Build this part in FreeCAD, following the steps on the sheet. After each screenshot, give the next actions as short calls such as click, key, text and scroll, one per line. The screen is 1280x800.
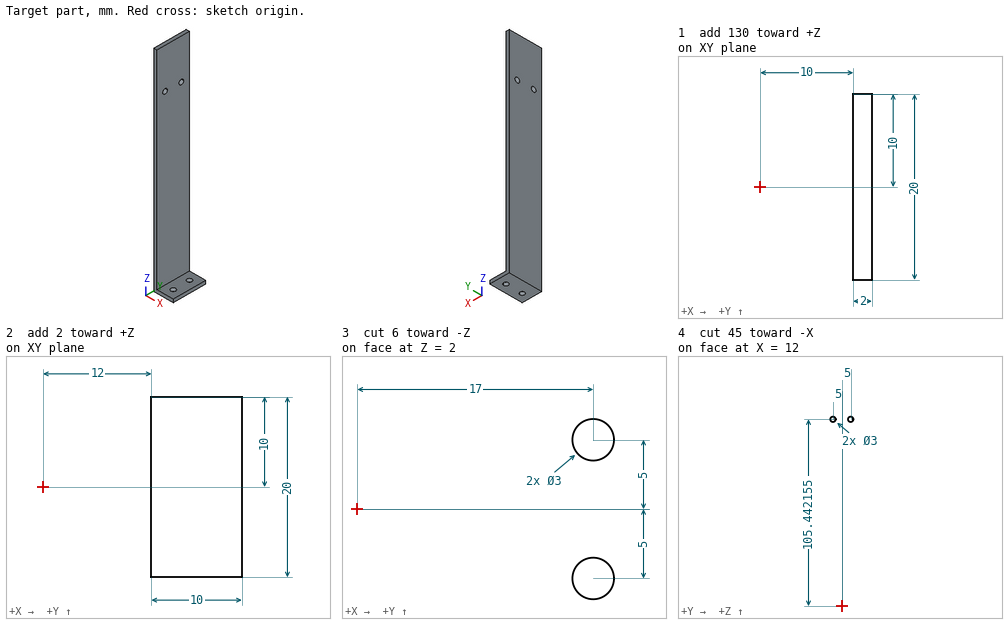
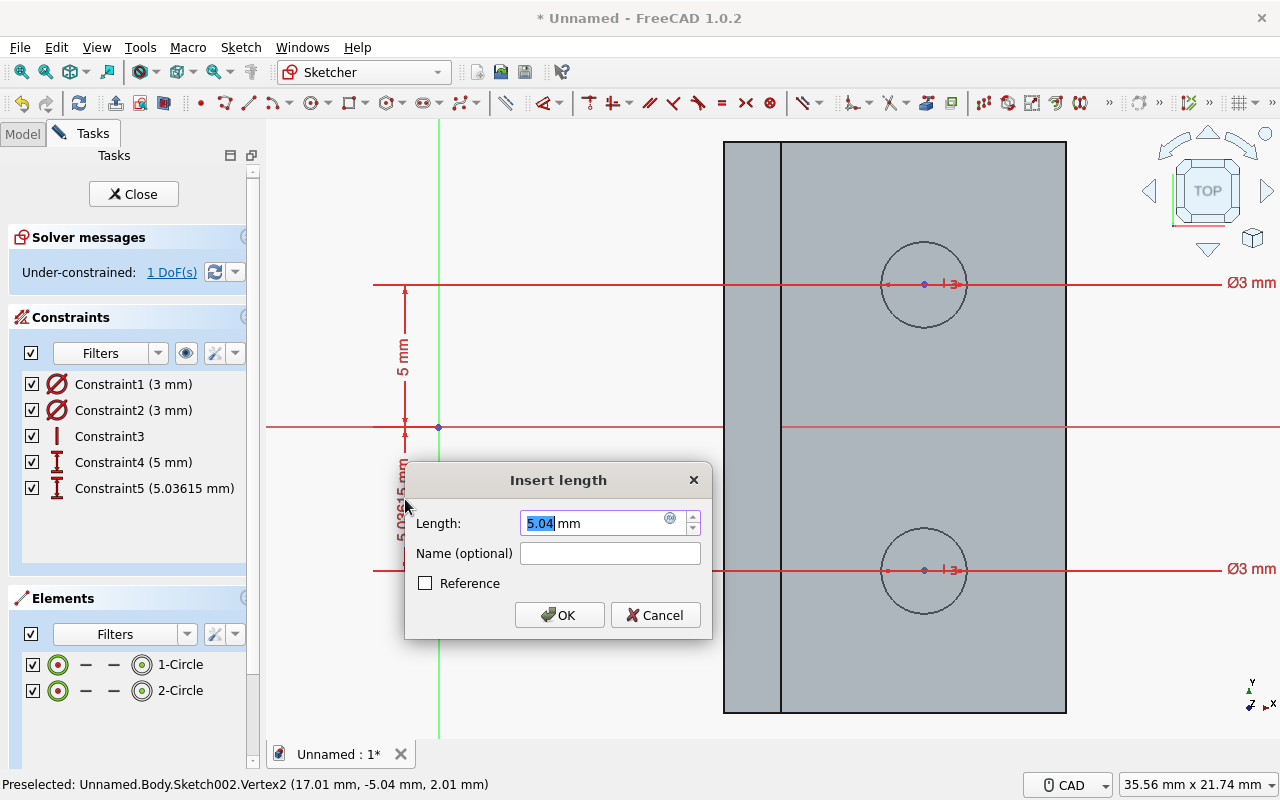
text(5)
key(Return)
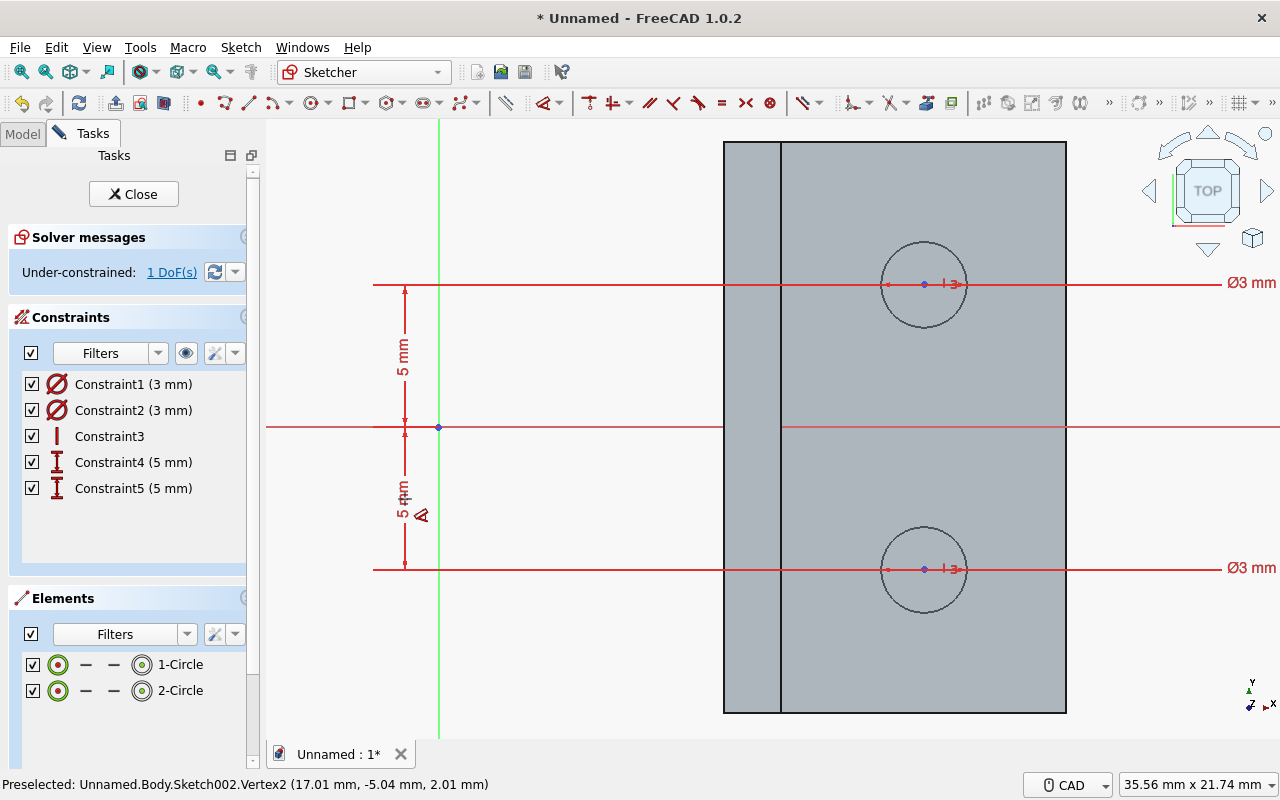
click(924, 285)
click(681, 251)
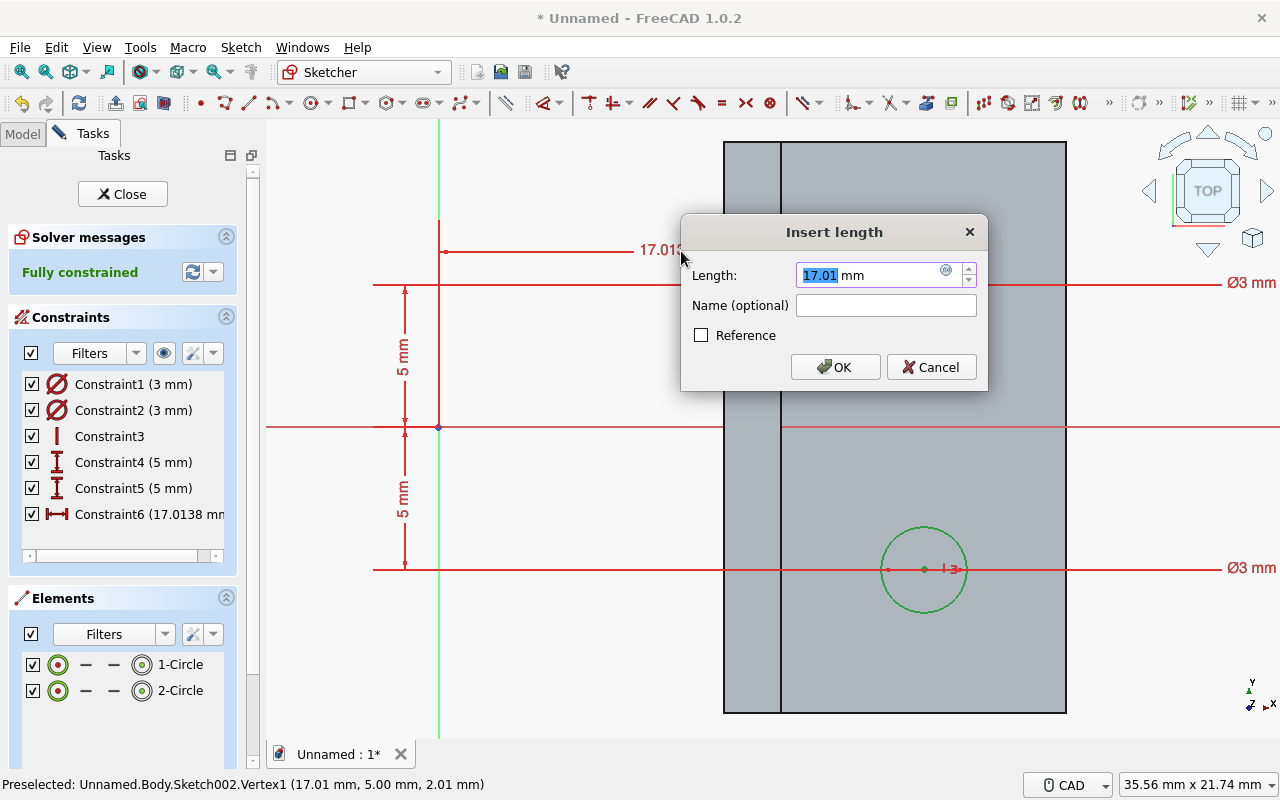
text(17)
key(Return)
key(Escape)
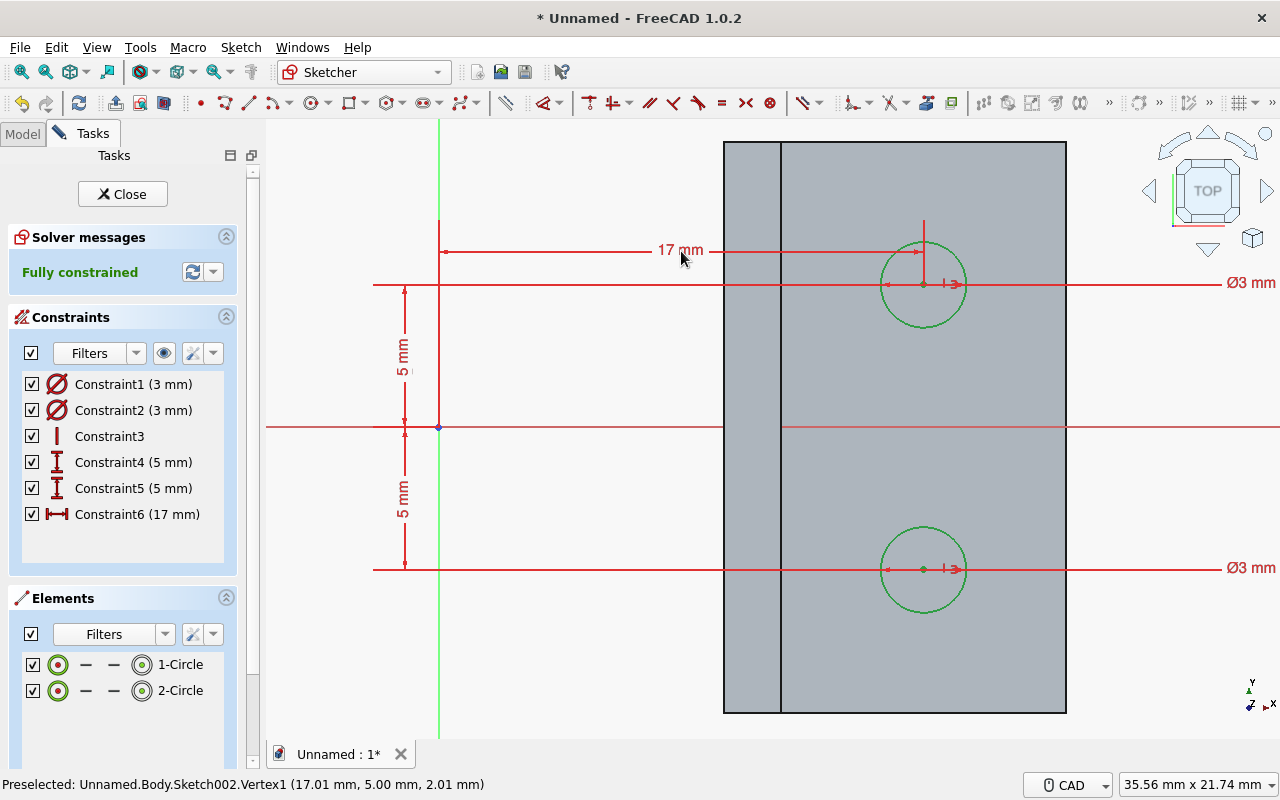
click(123, 194)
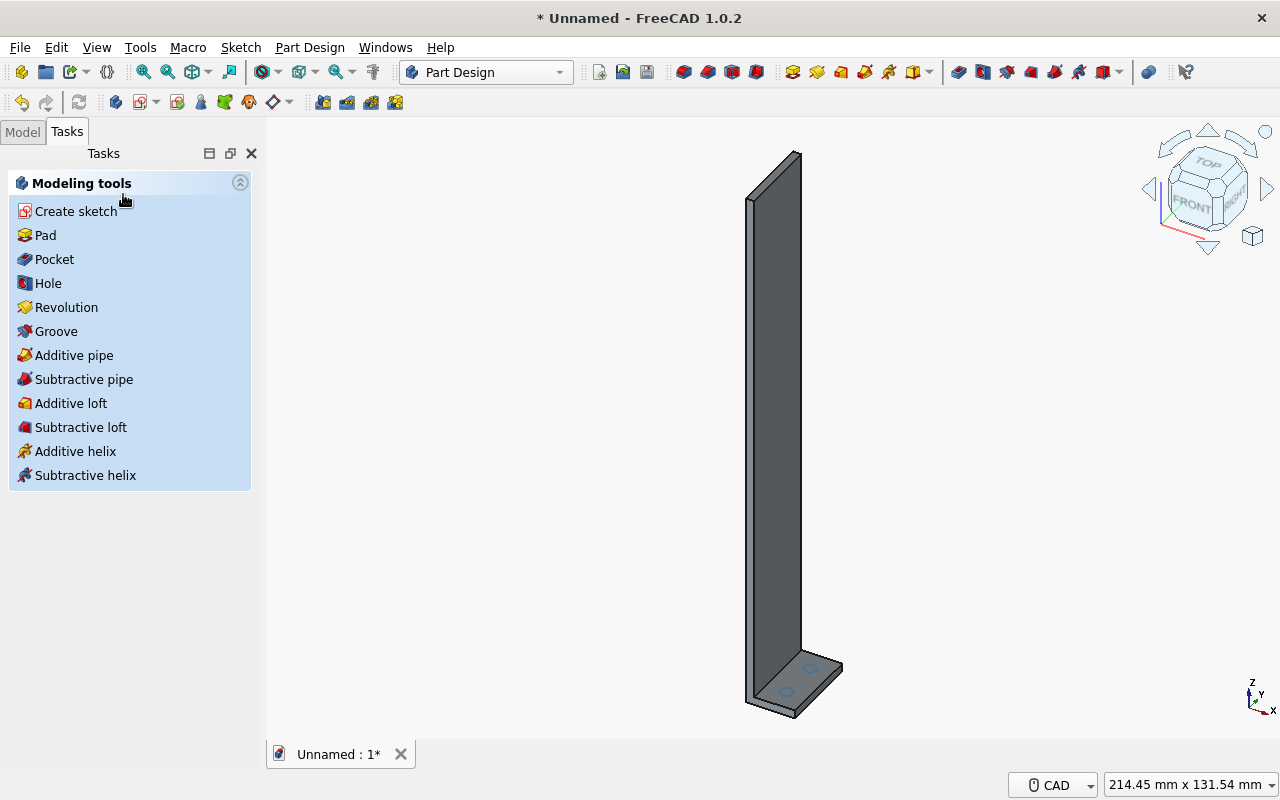
click(960, 72)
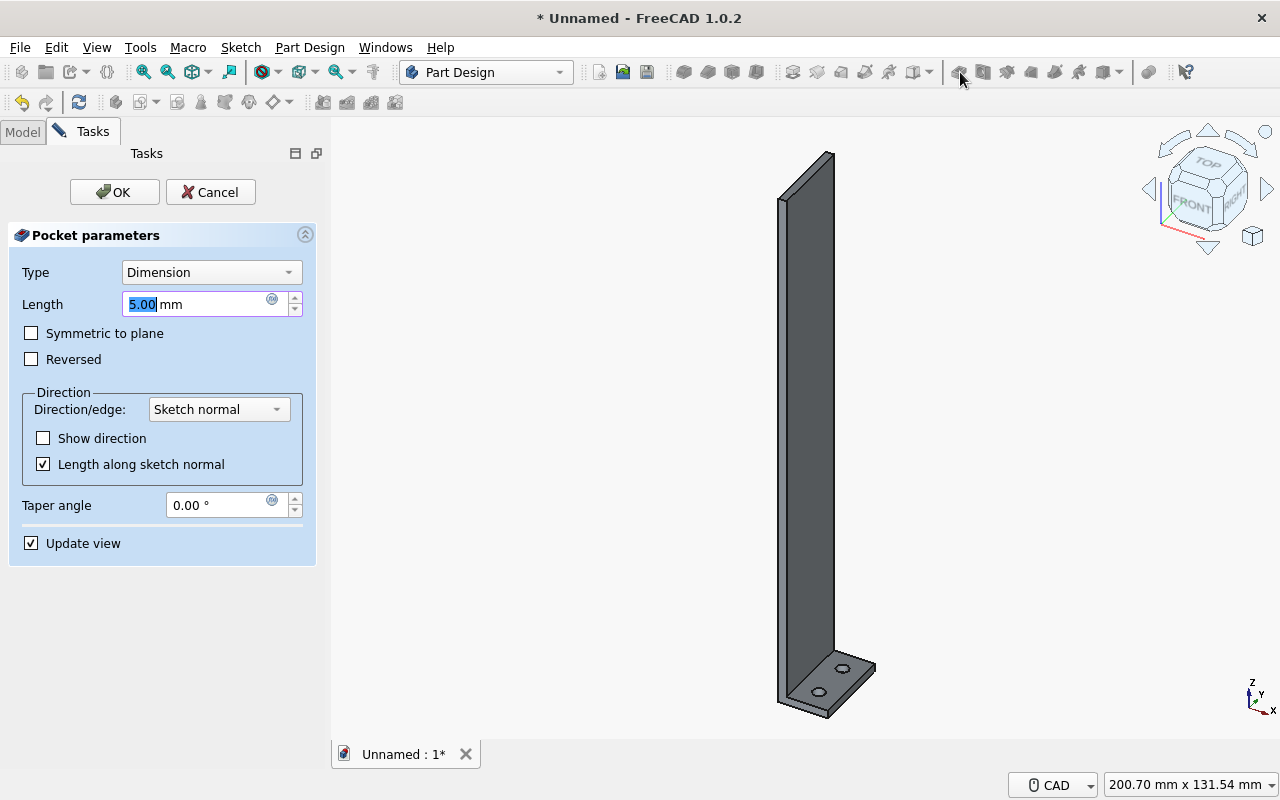
text(6)
key(Tab)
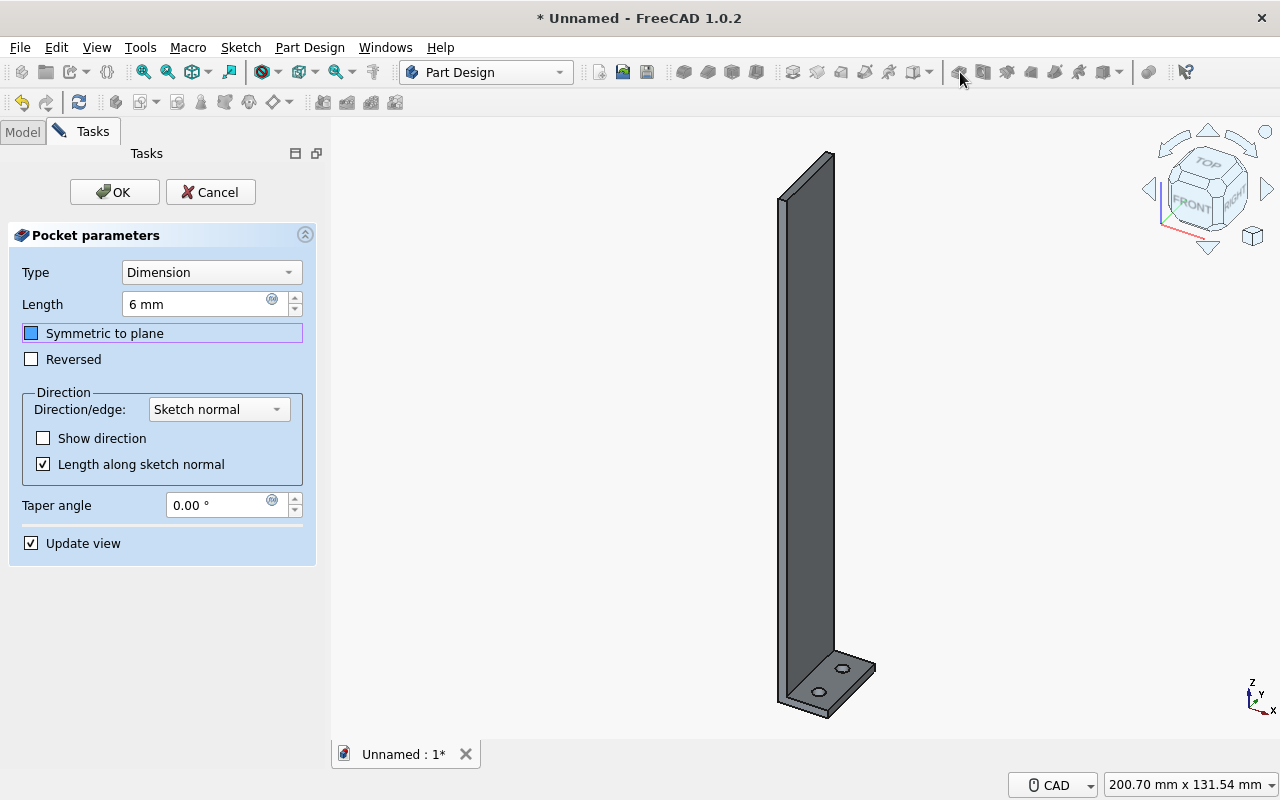
click(115, 192)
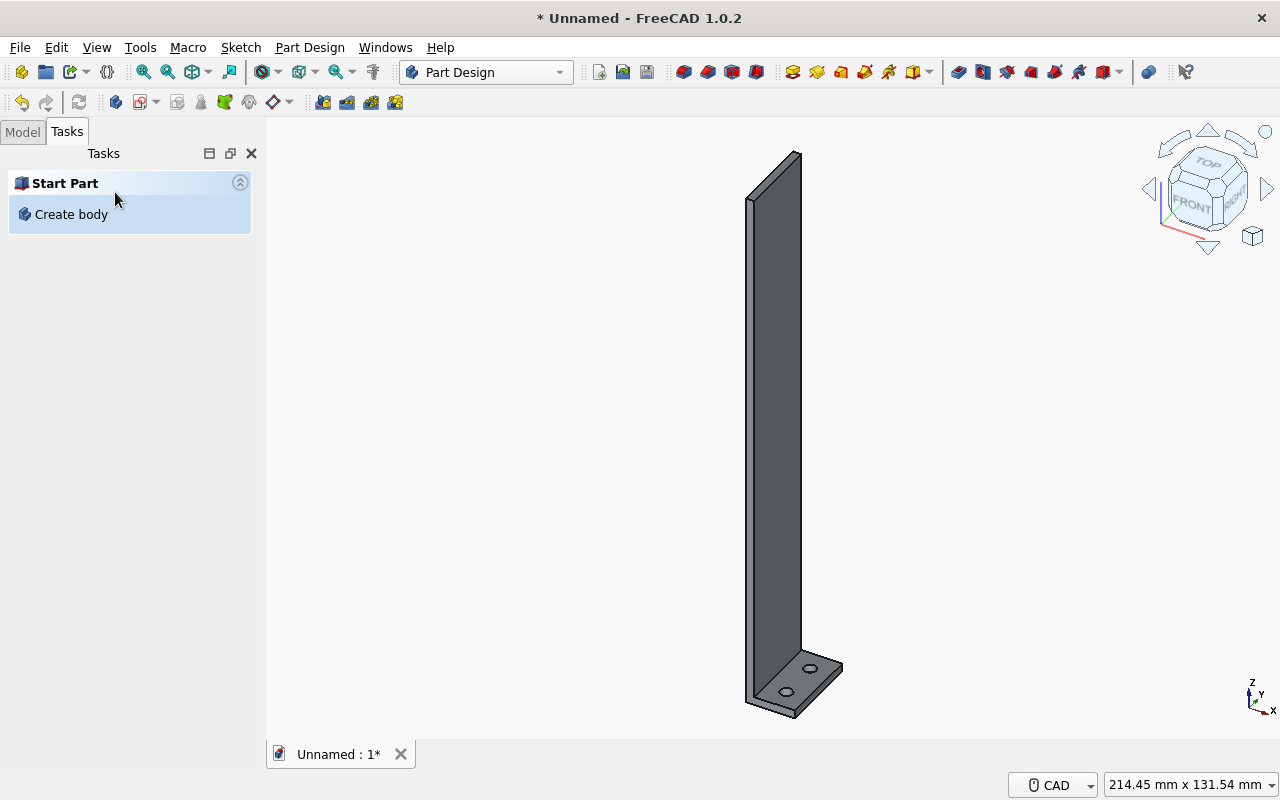
click(778, 283)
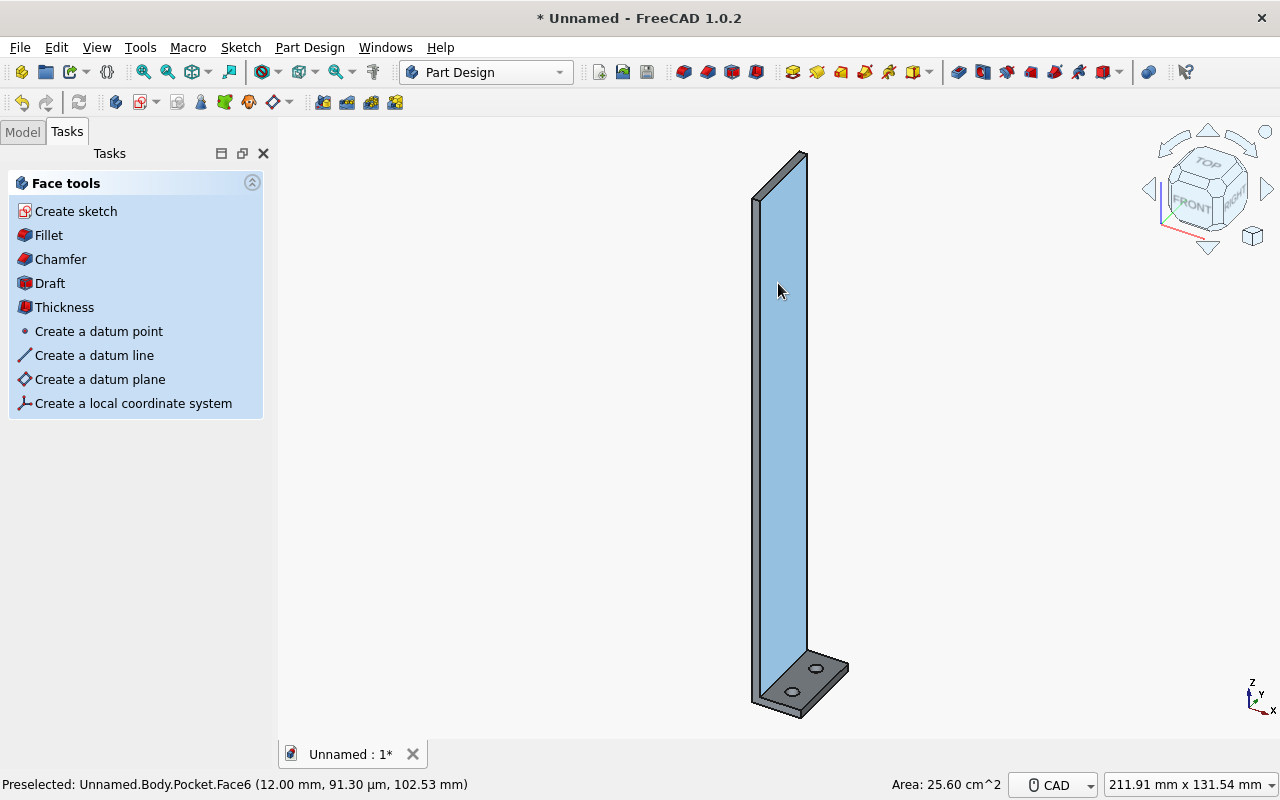
click(140, 102)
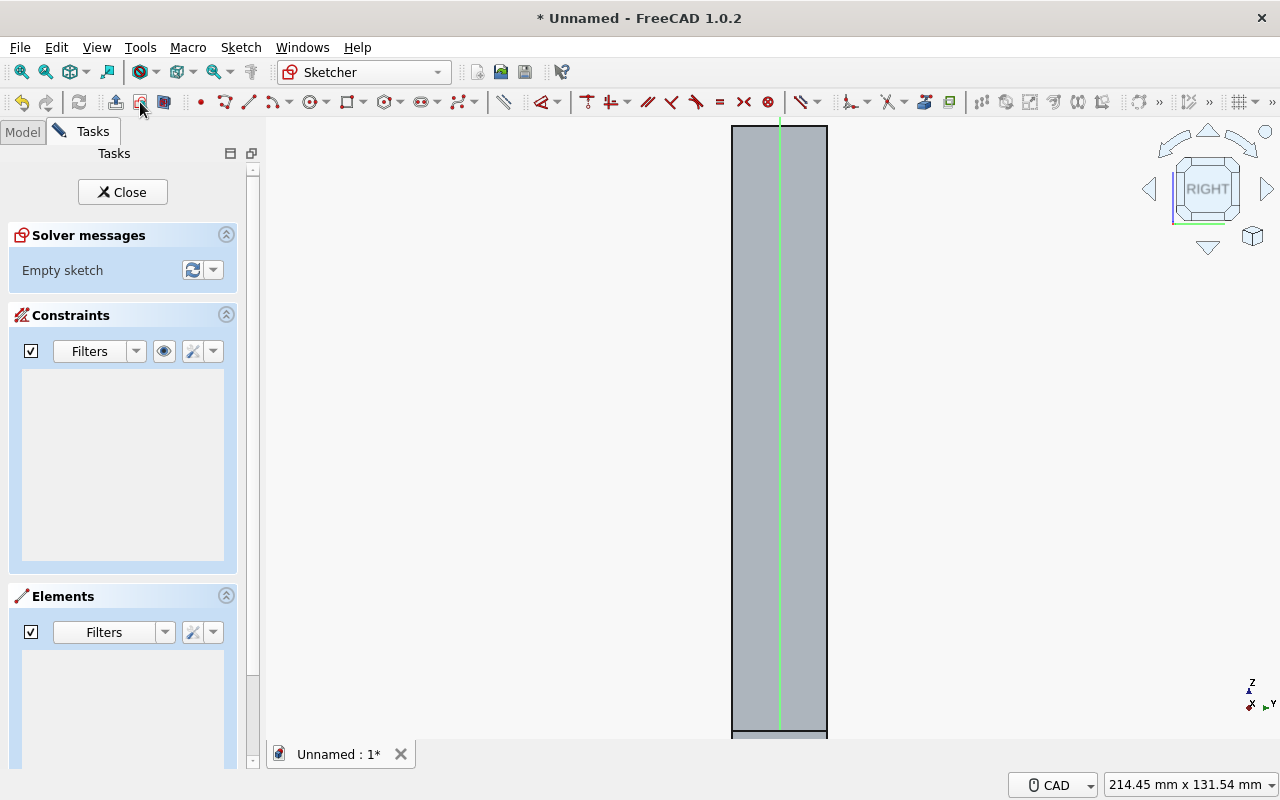
scroll(789, 219, up, 11)